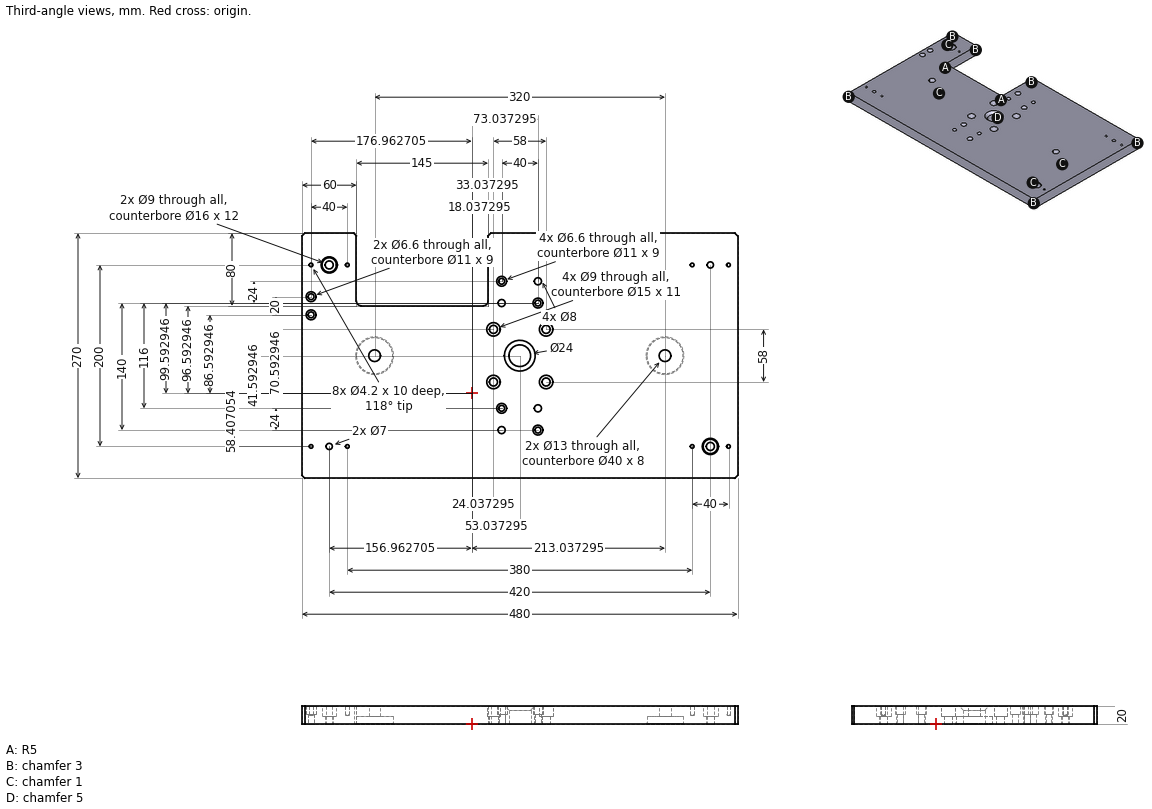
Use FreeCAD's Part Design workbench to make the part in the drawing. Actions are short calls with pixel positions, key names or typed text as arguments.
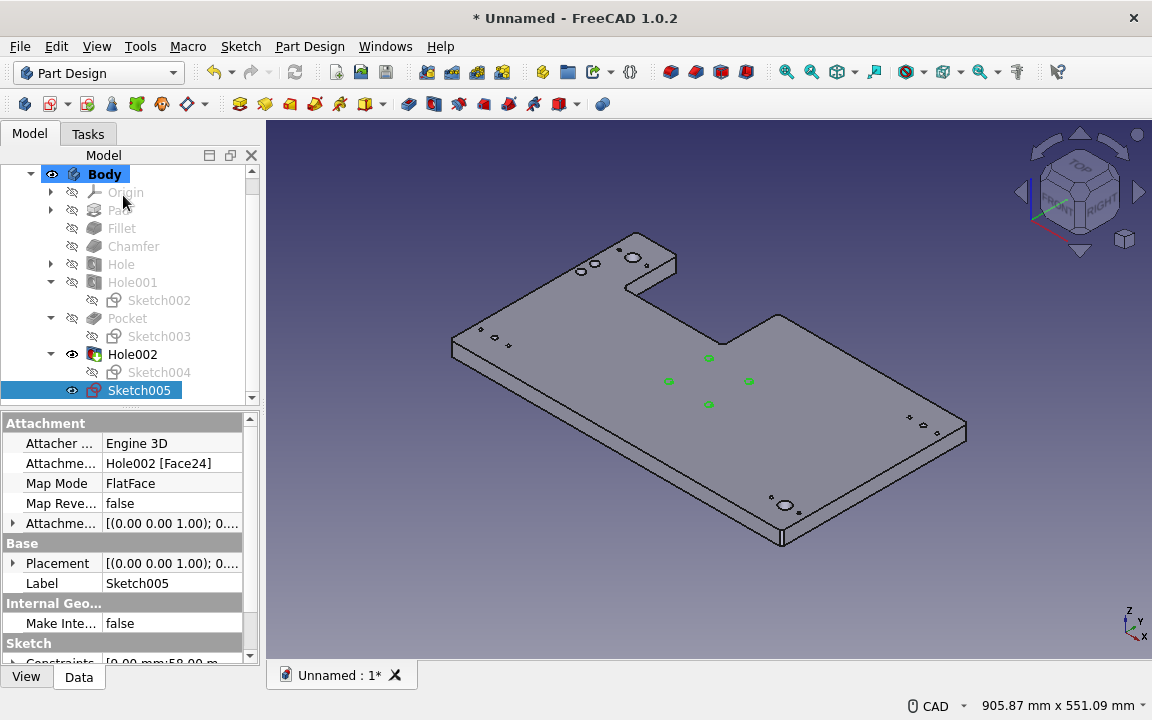
click(434, 104)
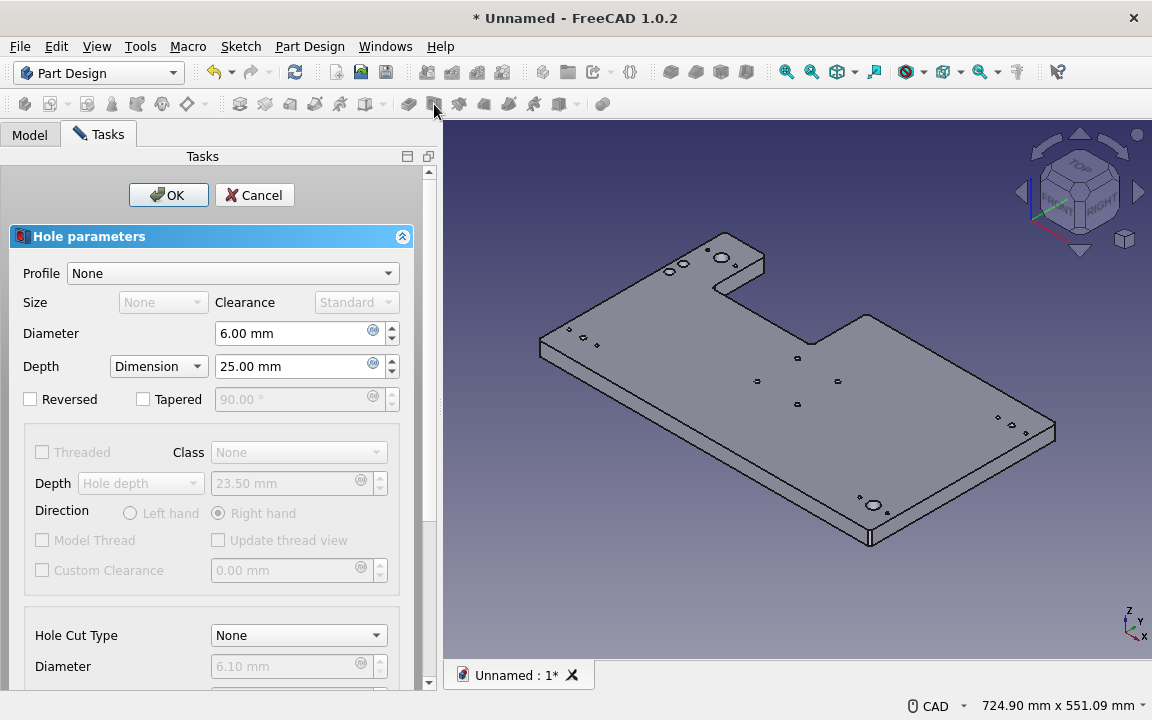
triple_click(300, 334)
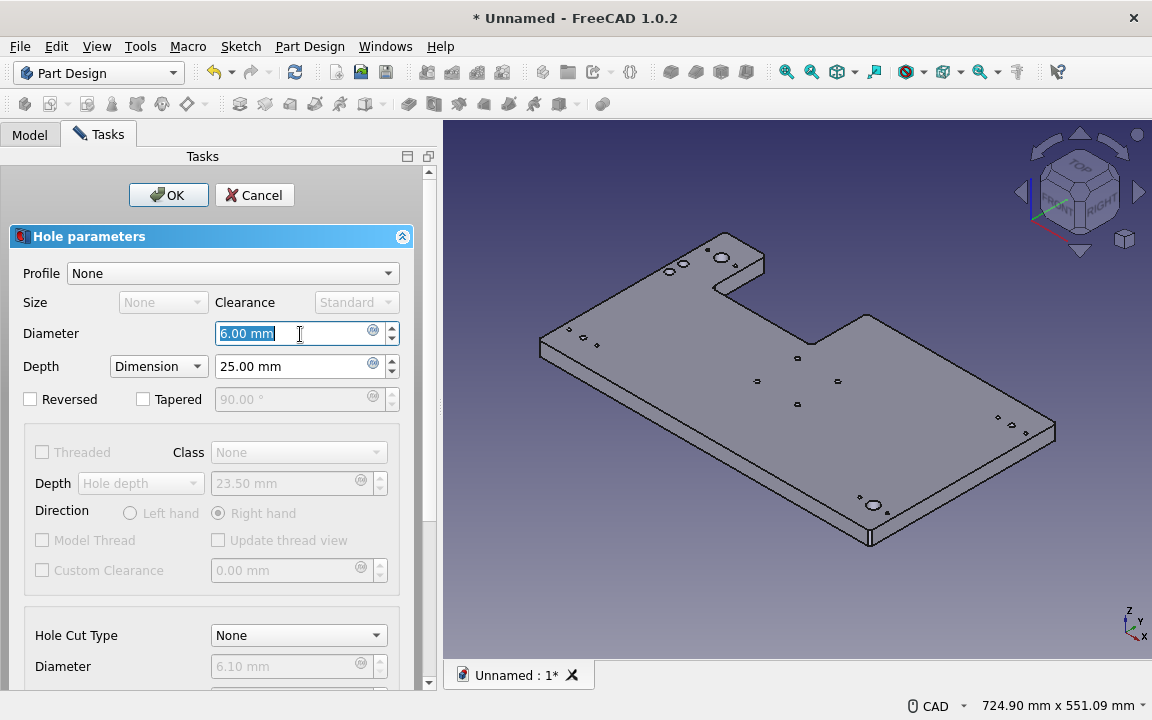
text(9)
key(Tab)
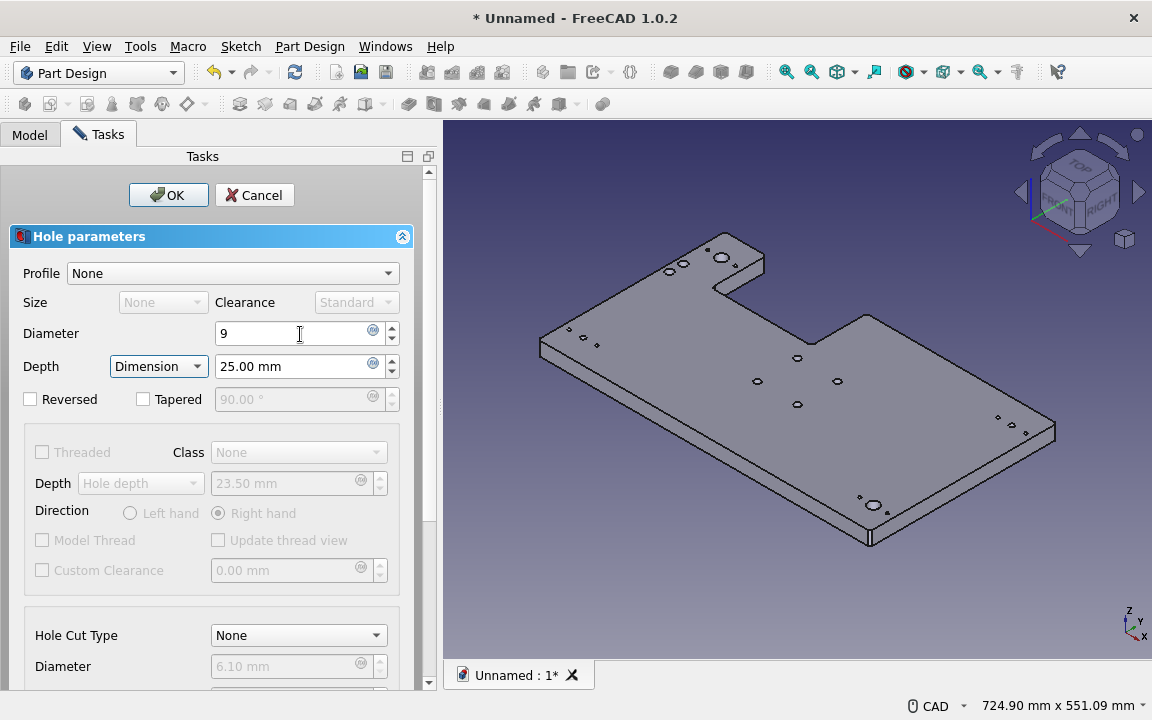
click(160, 366)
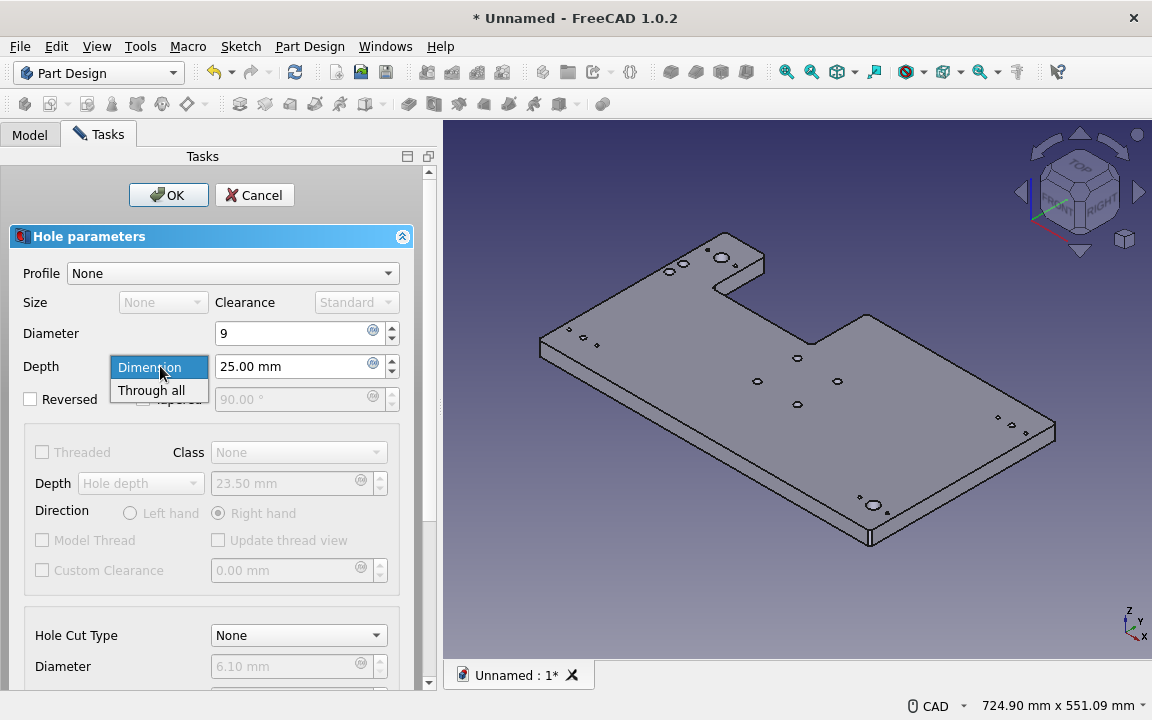
click(158, 390)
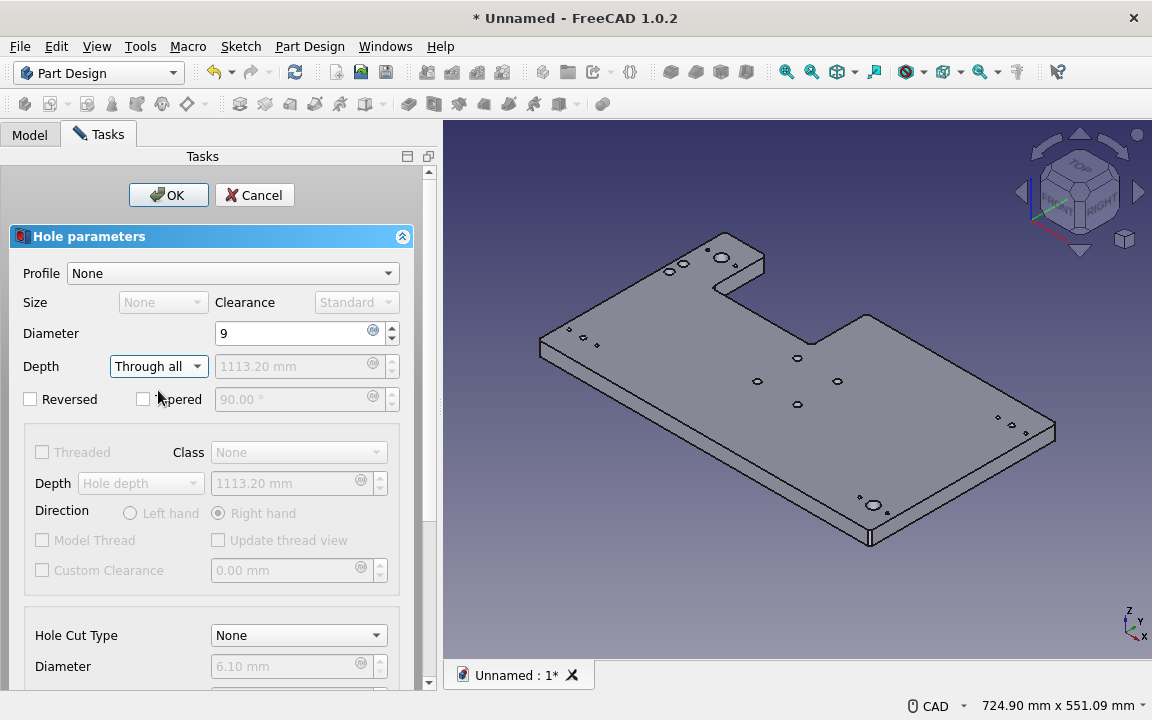
click(300, 636)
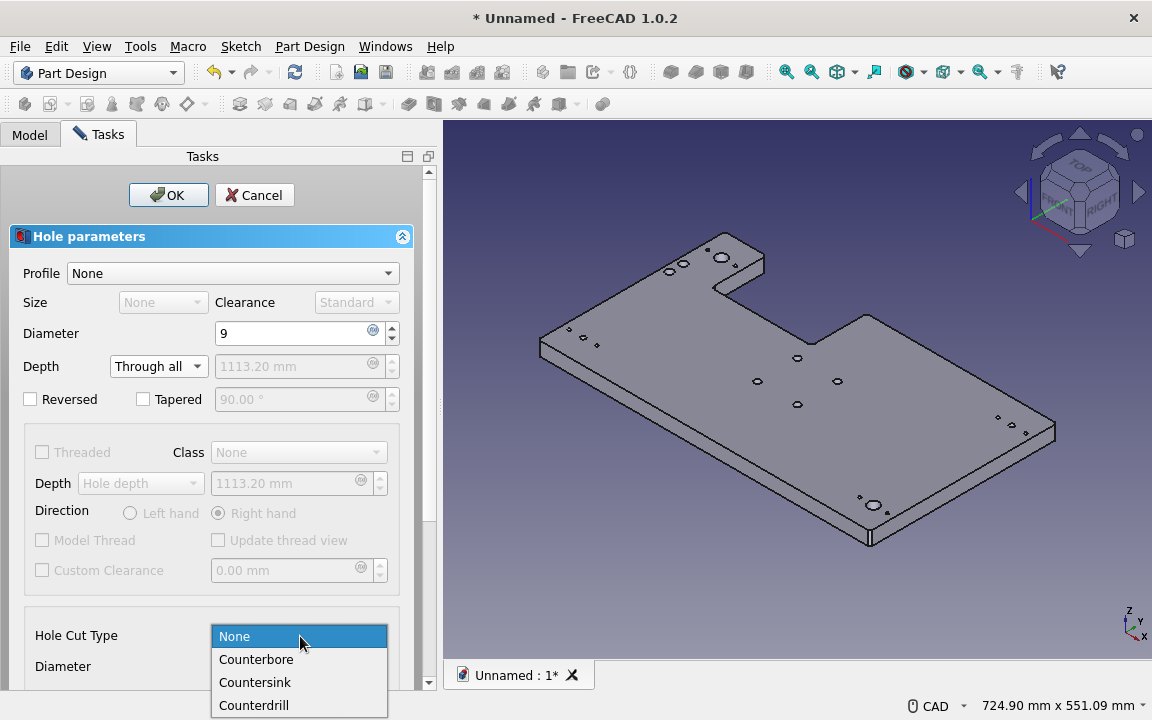
click(298, 660)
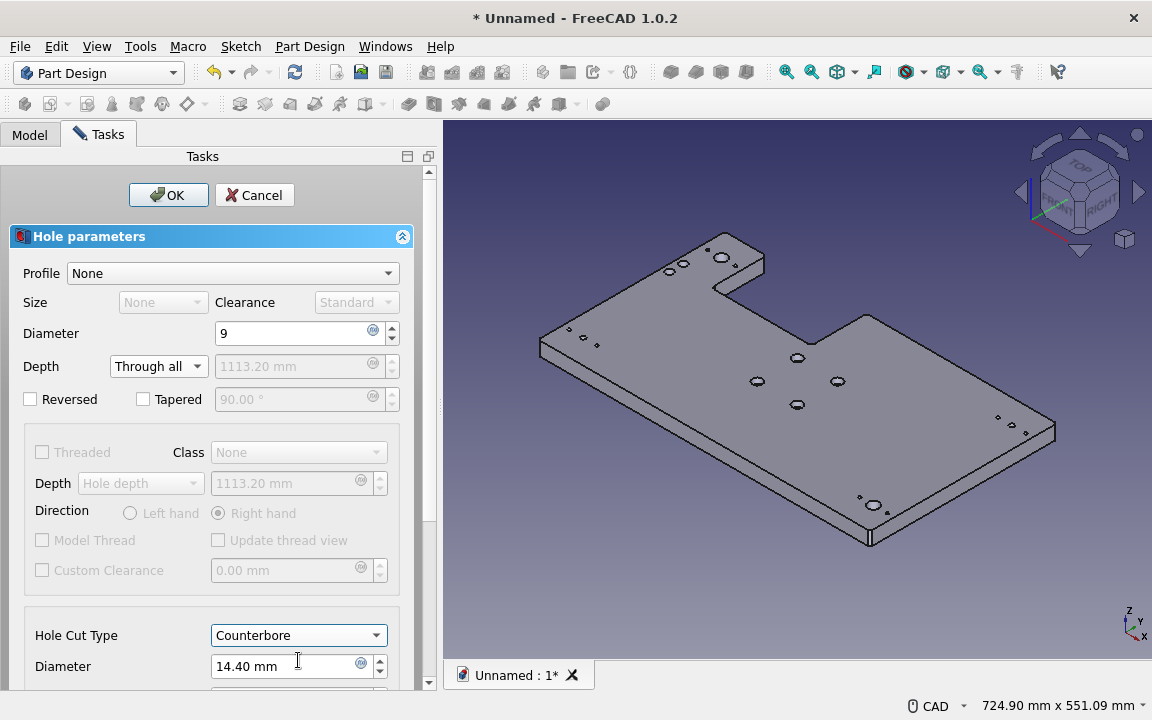
triple_click(292, 666)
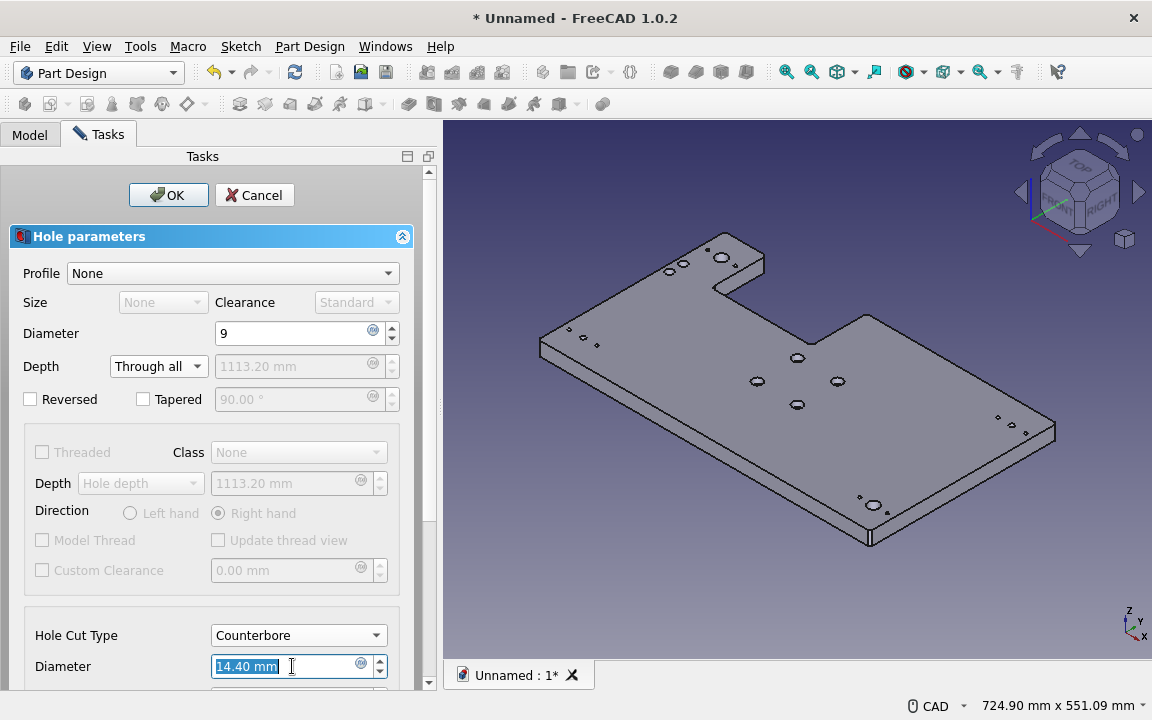
text(15)
key(Tab)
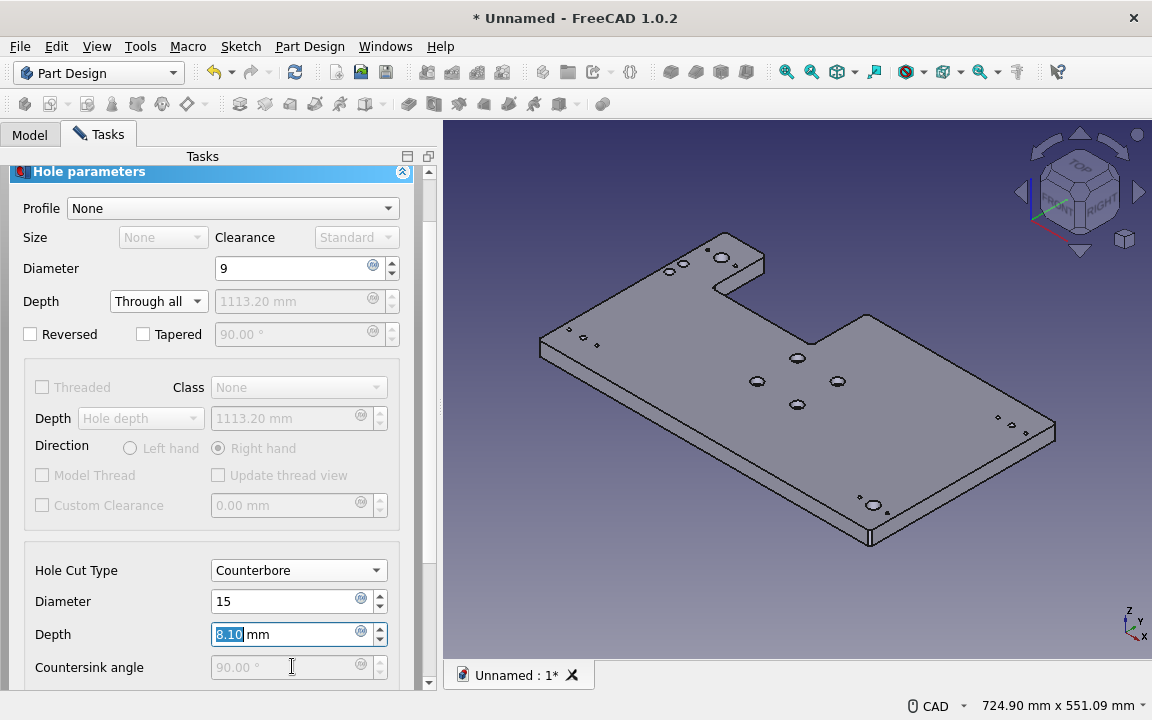
text(11)
key(Tab)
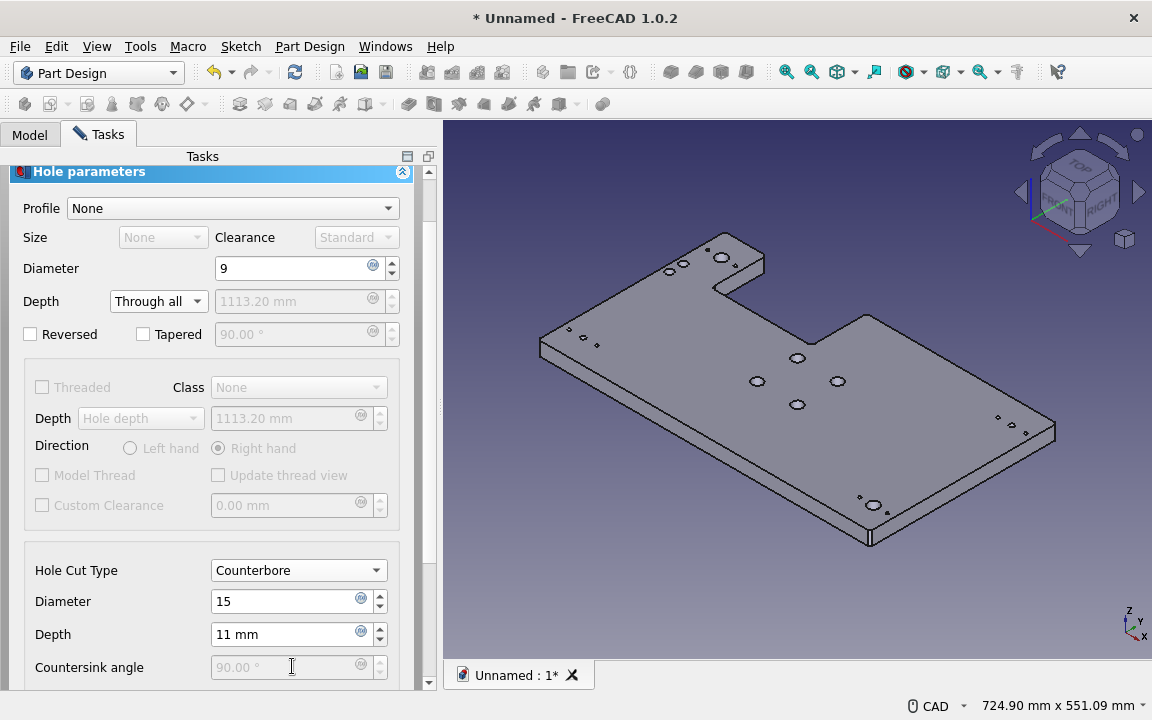
scroll(429, 428, up, 2)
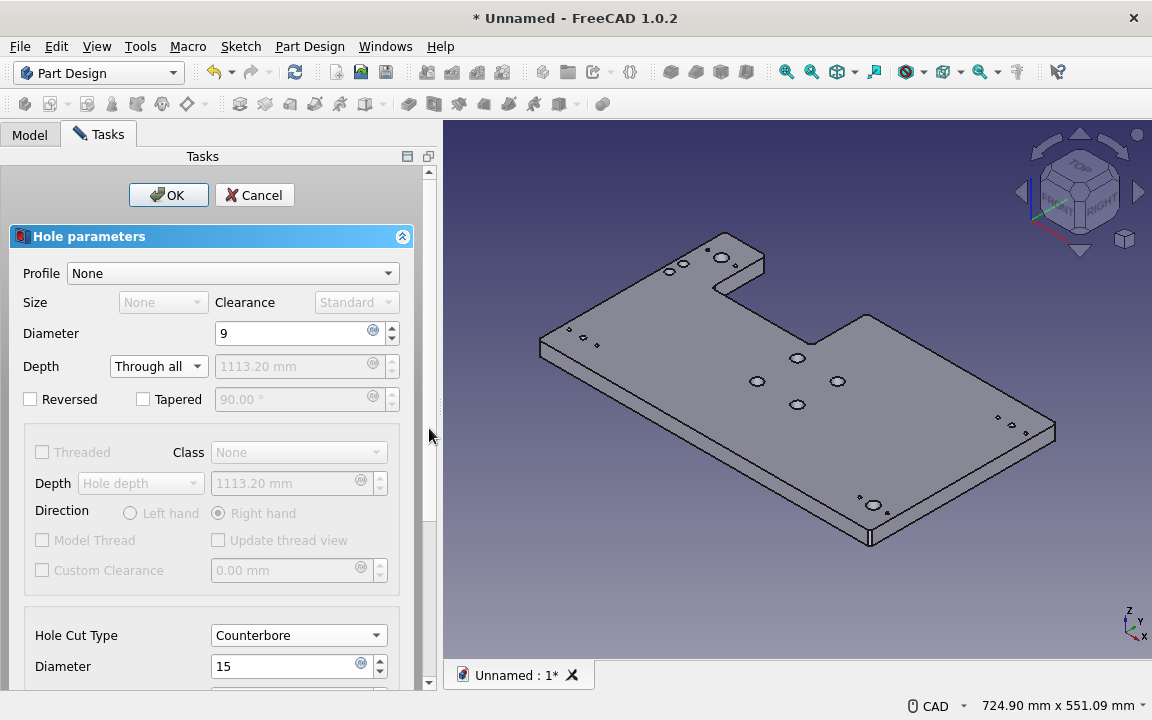
click(169, 195)